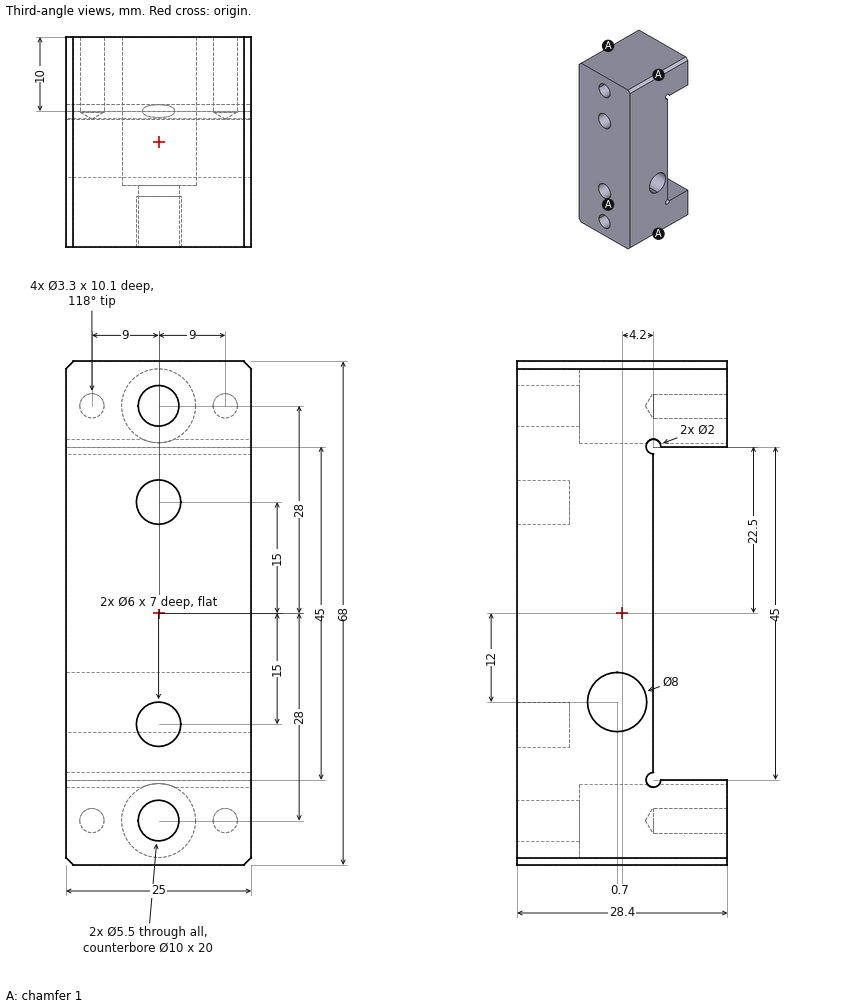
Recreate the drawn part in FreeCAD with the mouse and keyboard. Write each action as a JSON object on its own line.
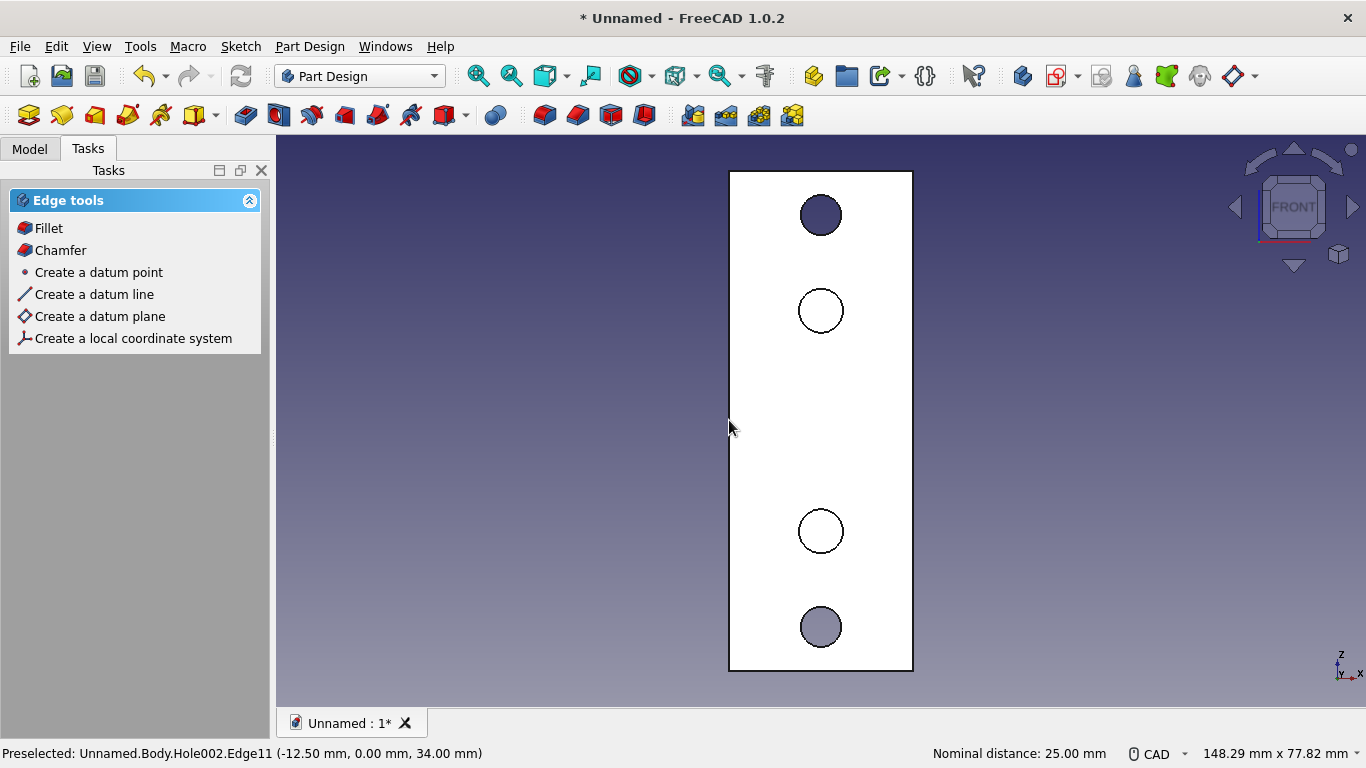
{"action": "key", "text": "3"}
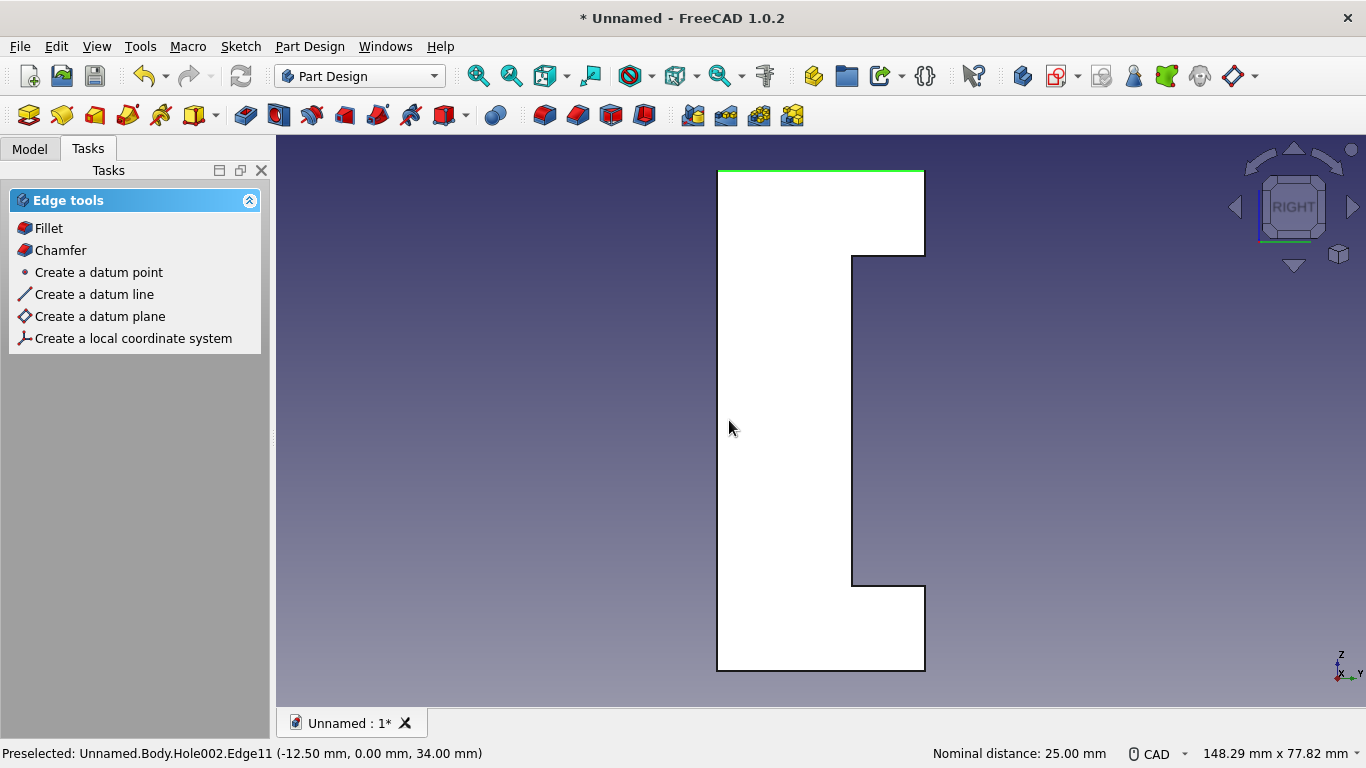
{"action": "left_click", "coordinate": [821, 670], "text": "ctrl"}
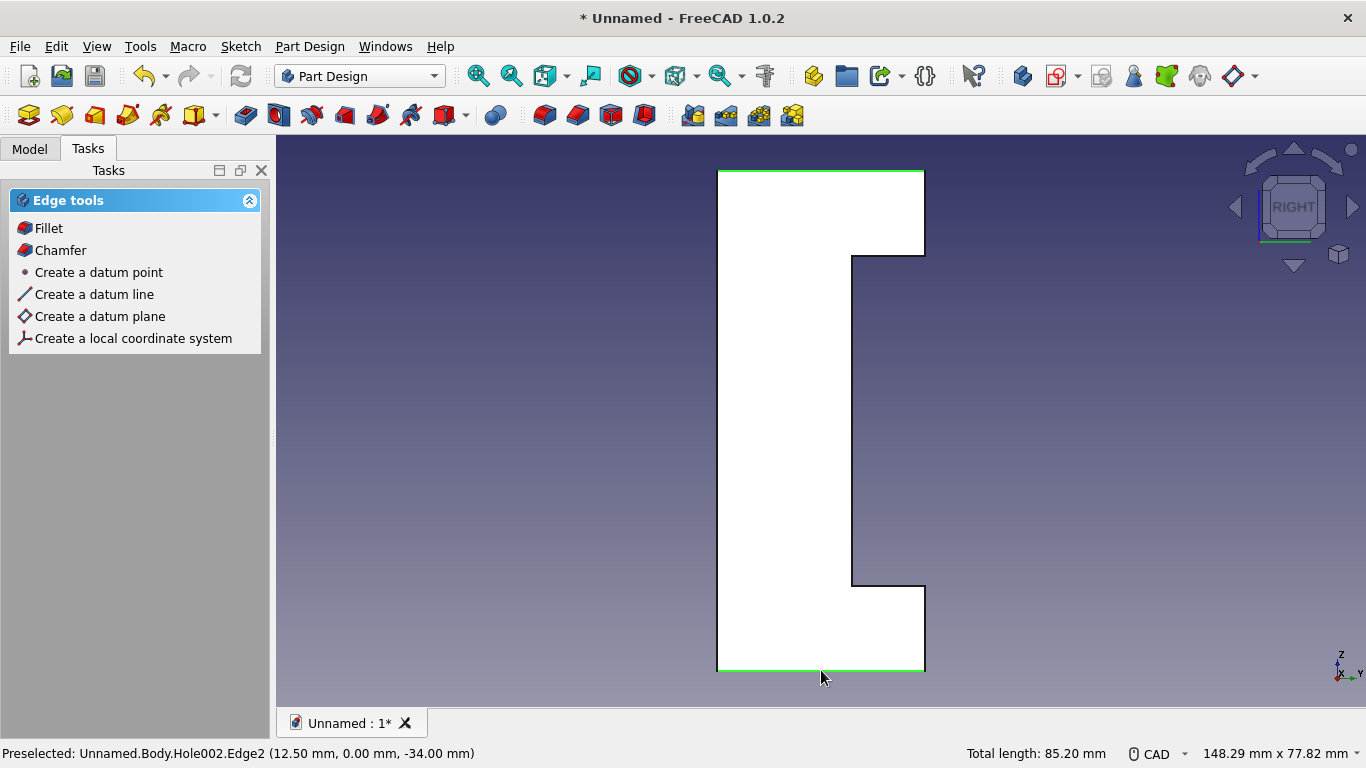
{"action": "key", "text": "5"}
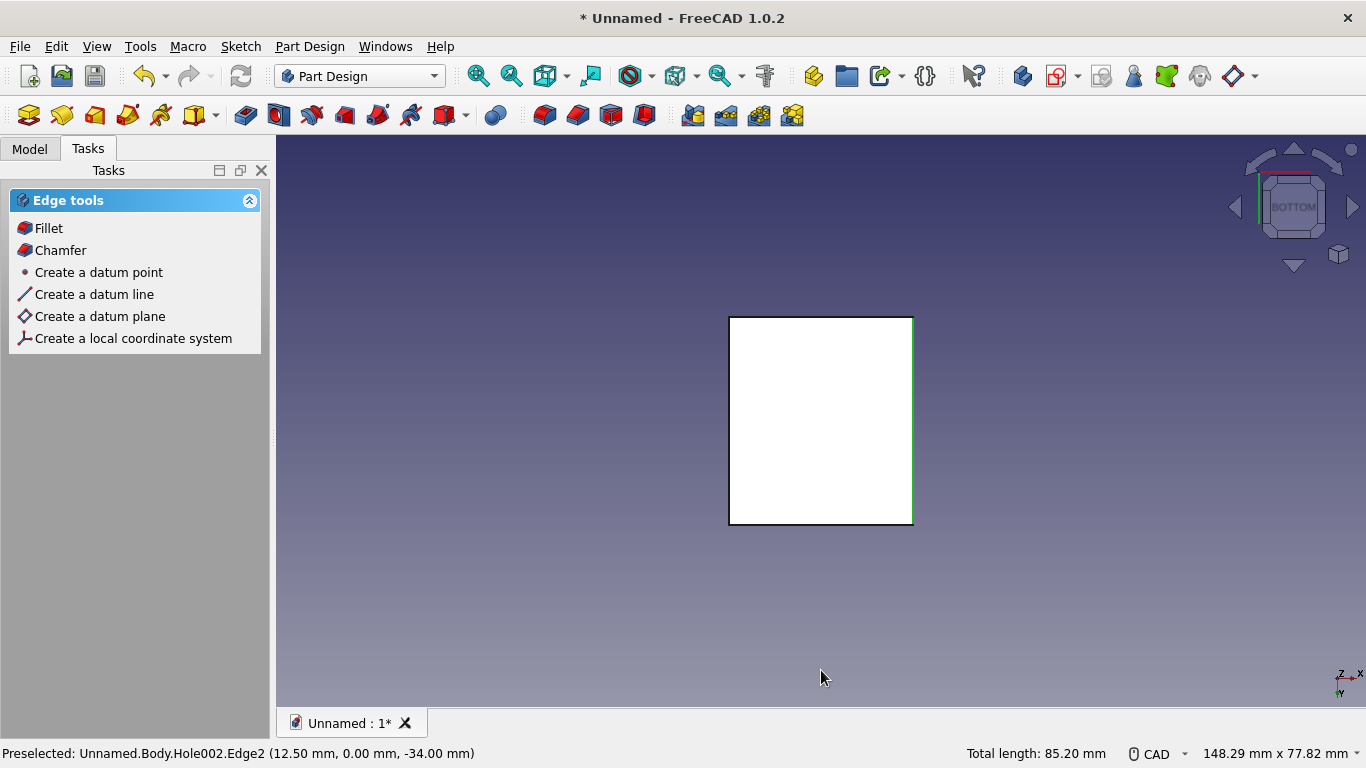
{"action": "key", "text": "v f"}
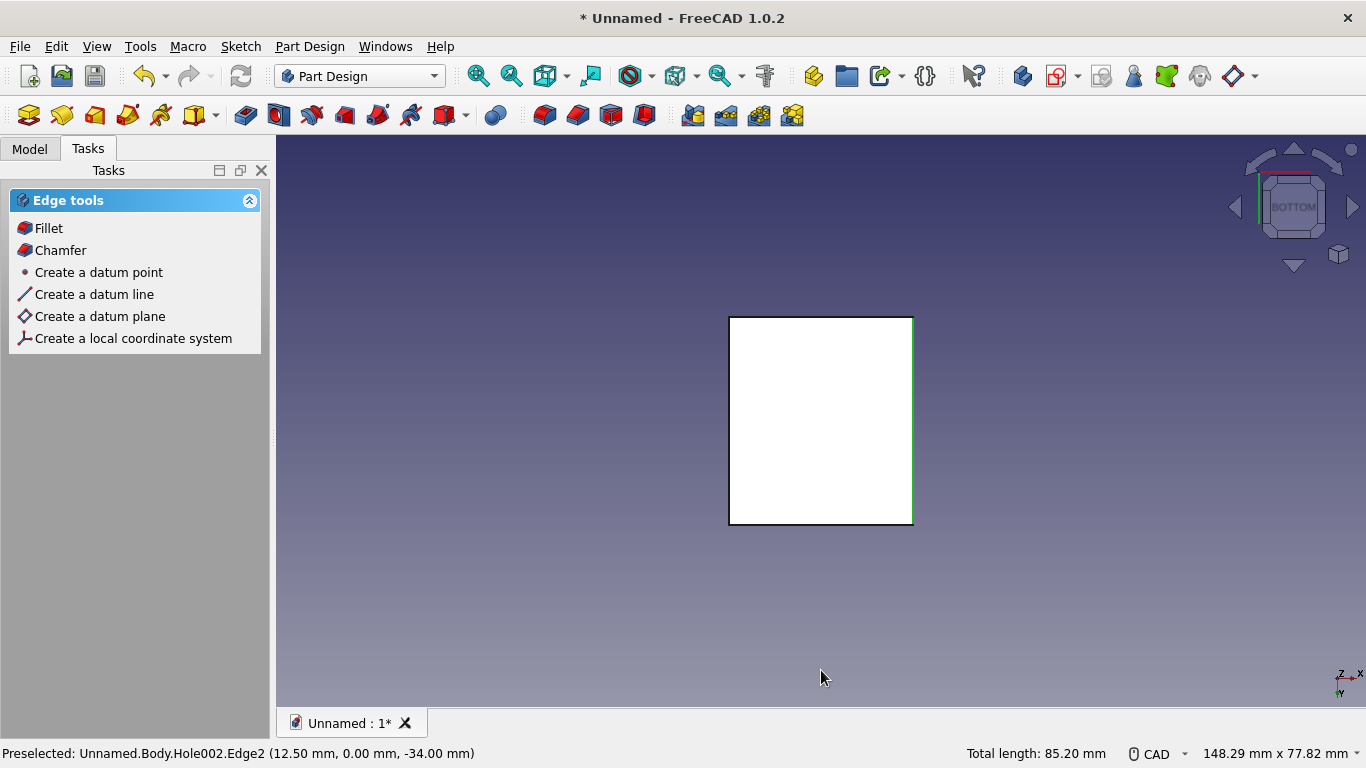
{"action": "left_click", "coordinate": [729, 420], "text": "ctrl"}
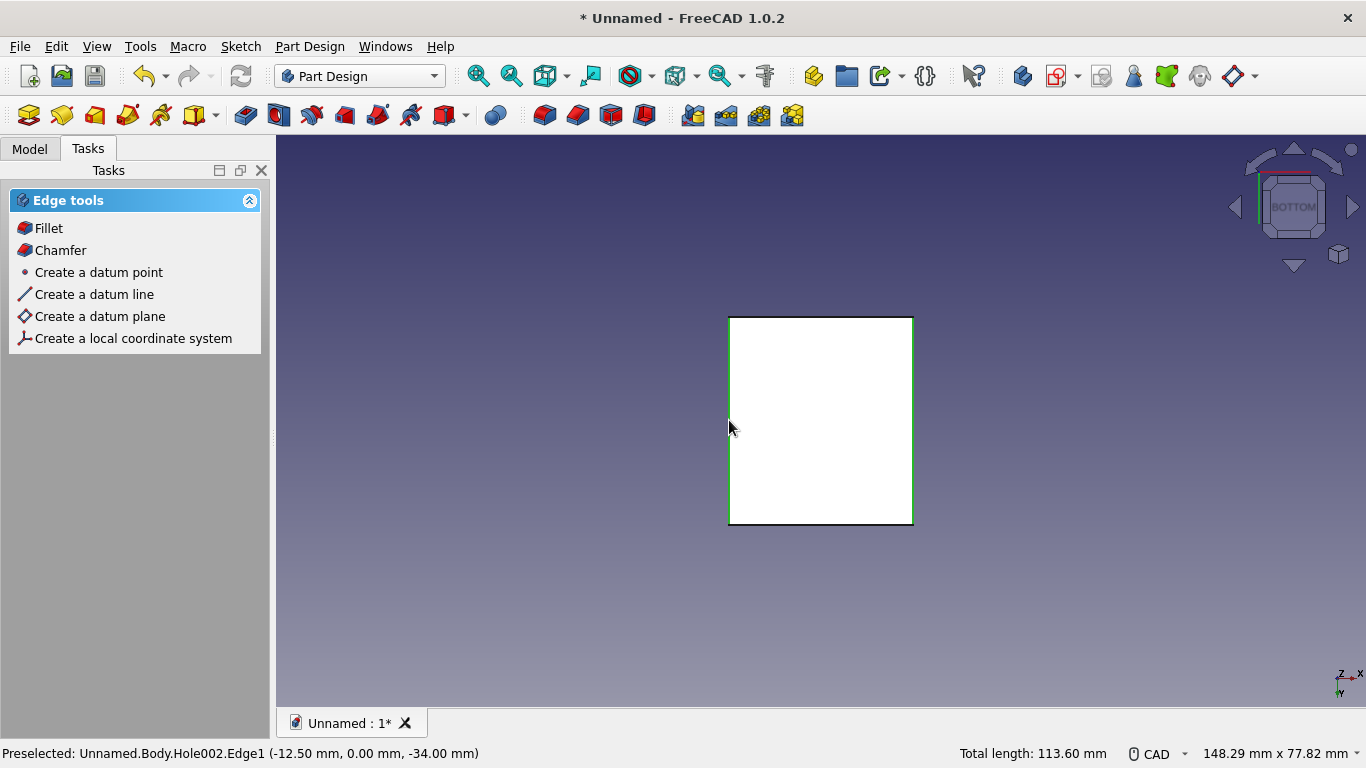
{"action": "left_click", "coordinate": [578, 116]}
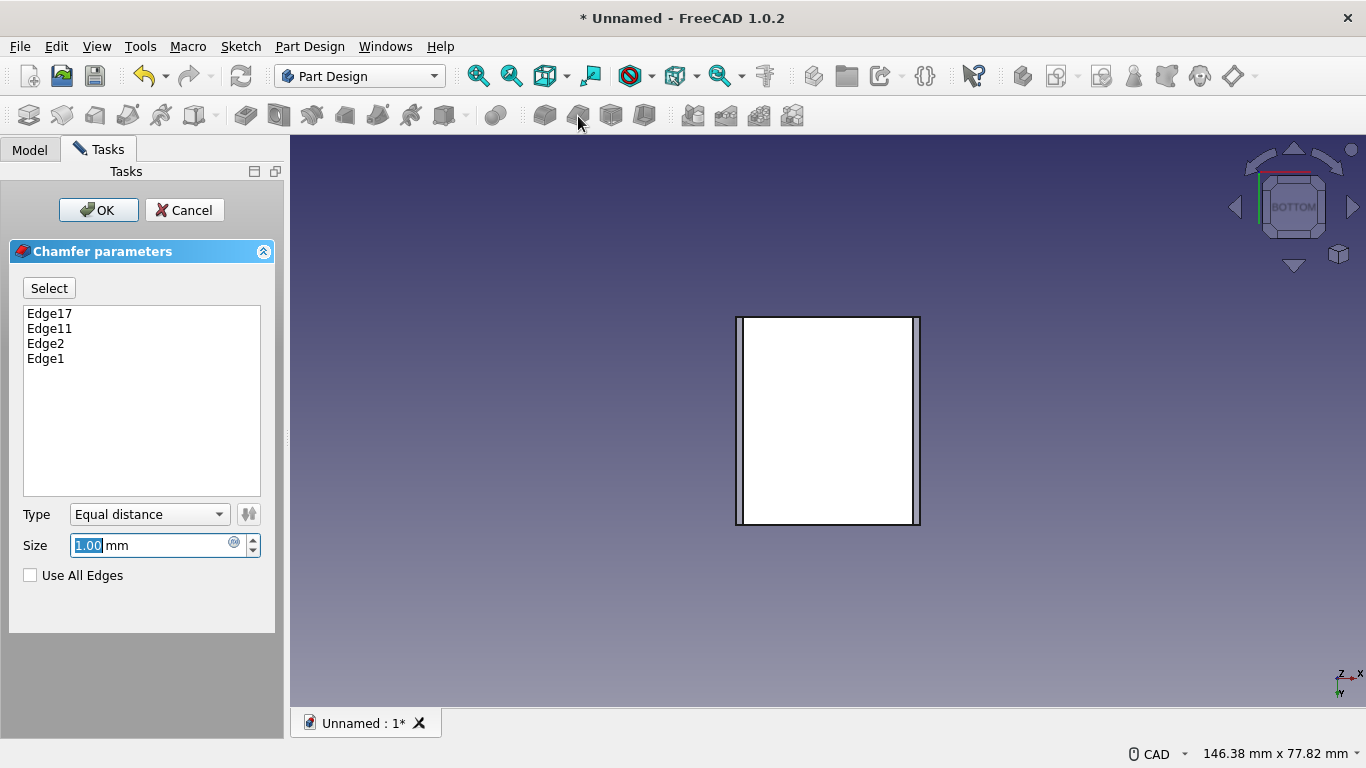
{"action": "type", "text": "1"}
{"action": "key", "text": "Tab"}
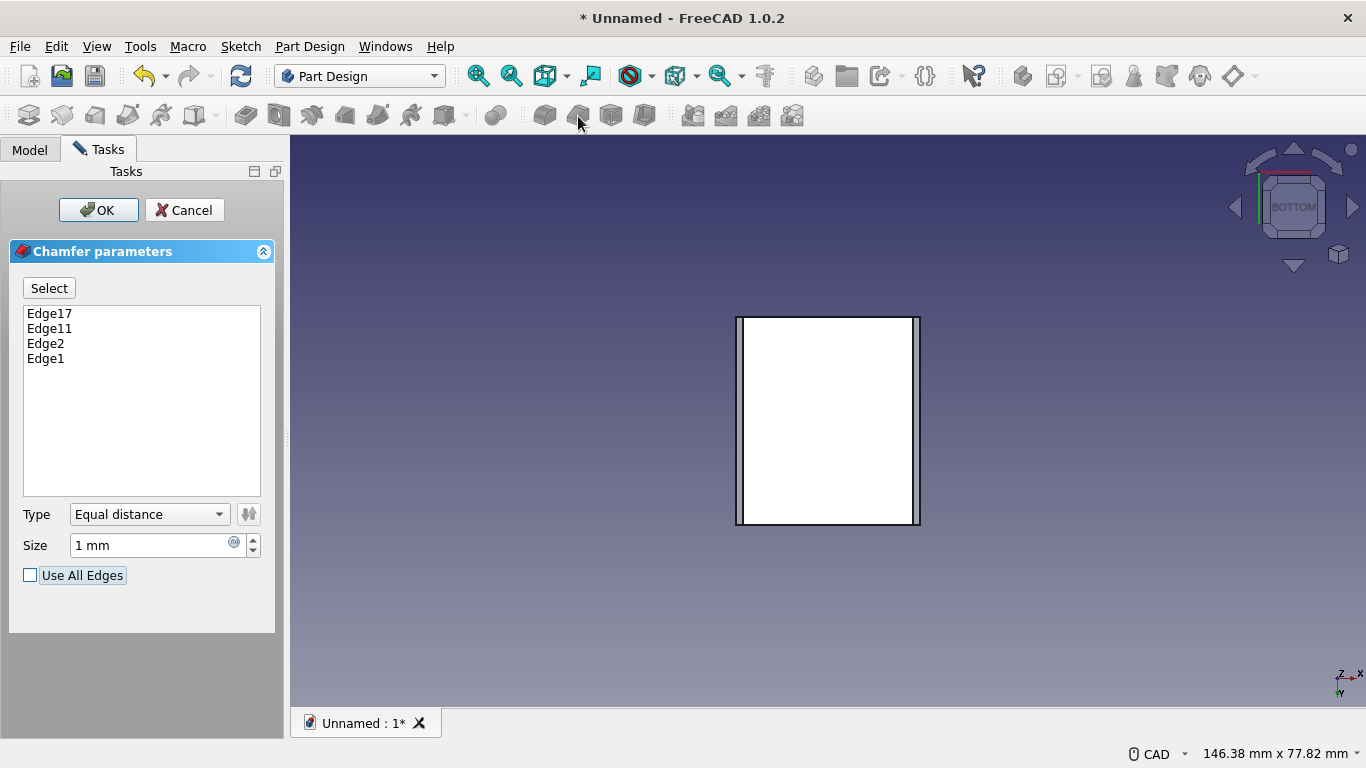
{"action": "left_click", "coordinate": [99, 210]}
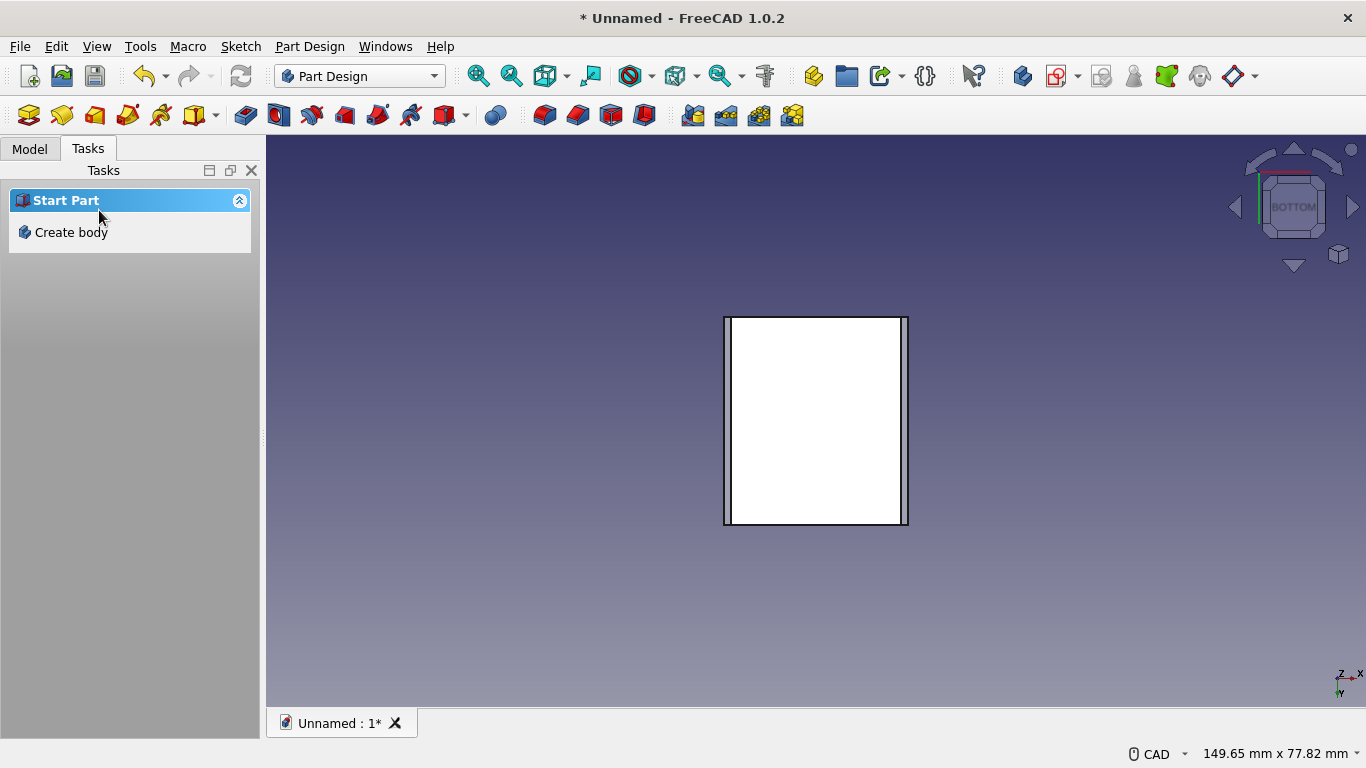
{"action": "key", "text": "v f"}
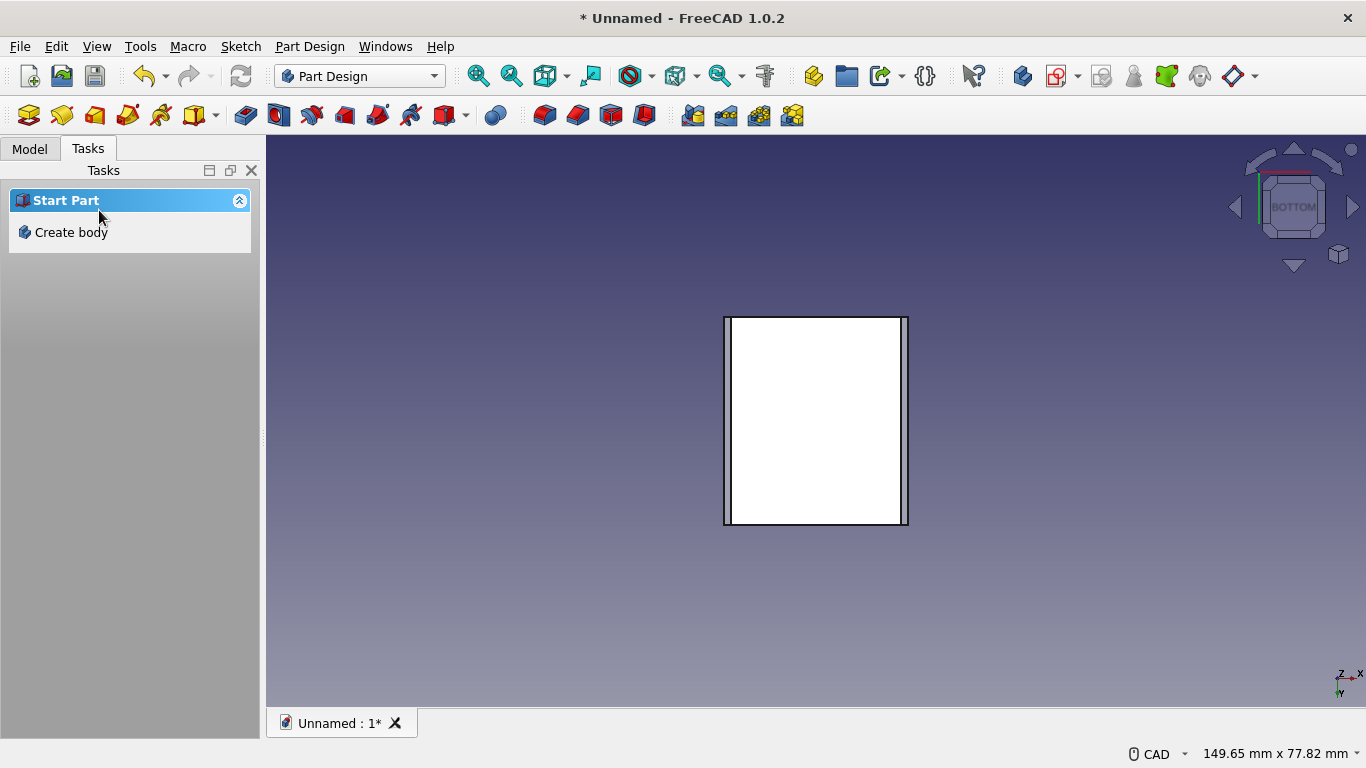
{"action": "key", "text": "6"}